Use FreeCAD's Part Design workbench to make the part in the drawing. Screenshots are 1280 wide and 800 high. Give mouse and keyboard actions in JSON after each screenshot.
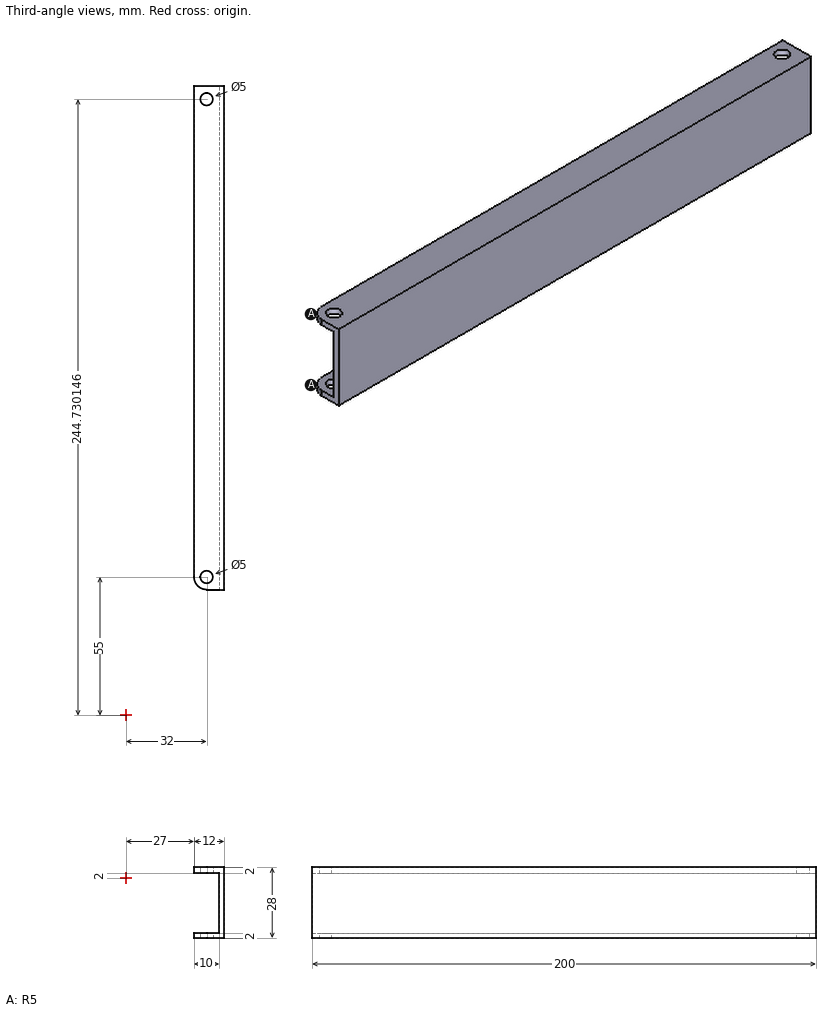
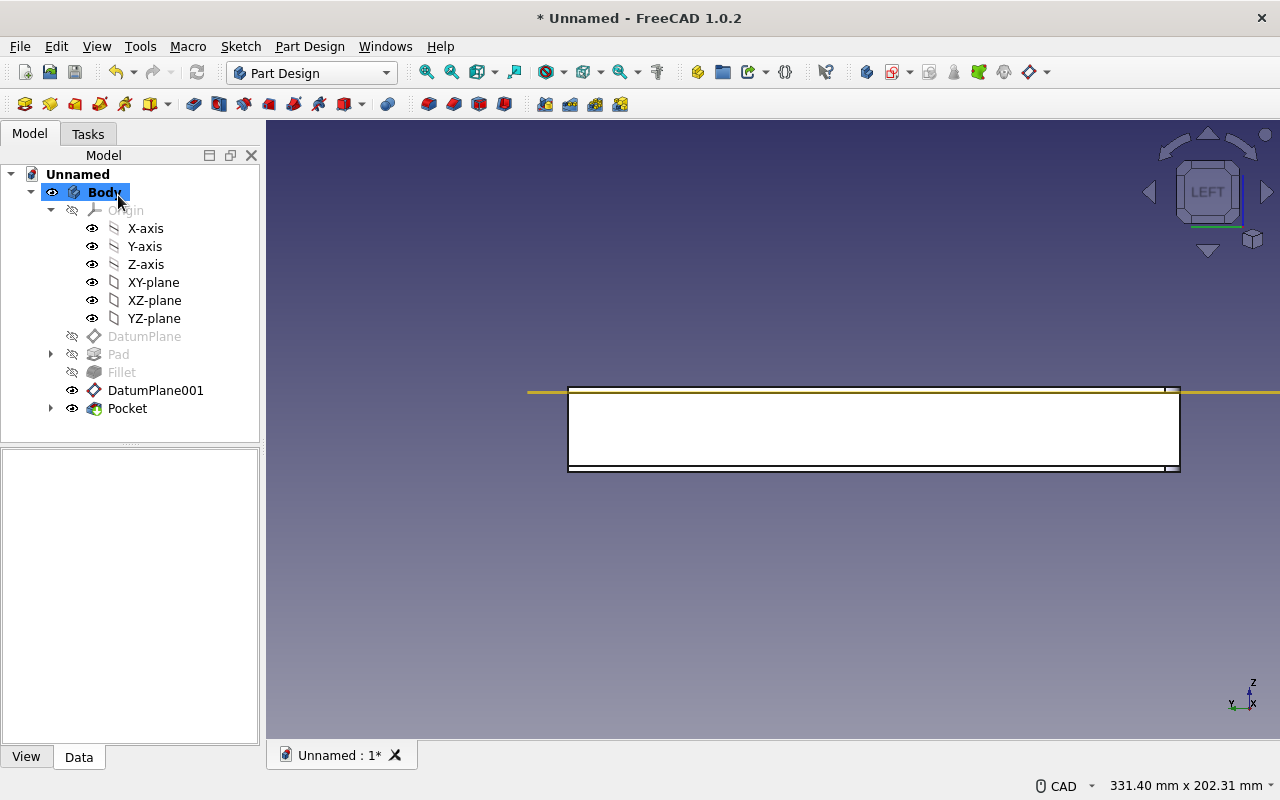
{"action": "left_click", "coordinate": [117, 390]}
{"action": "key", "text": "space"}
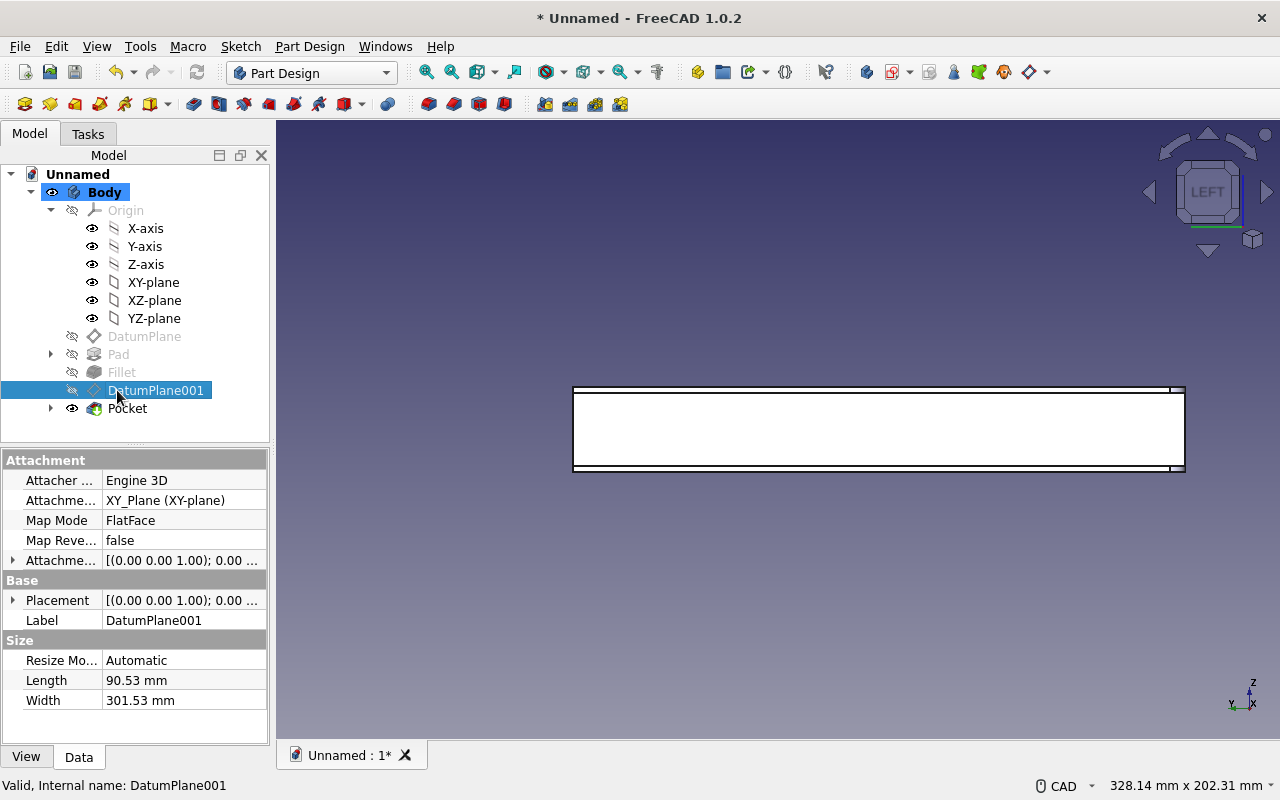
{"action": "left_click", "coordinate": [137, 282]}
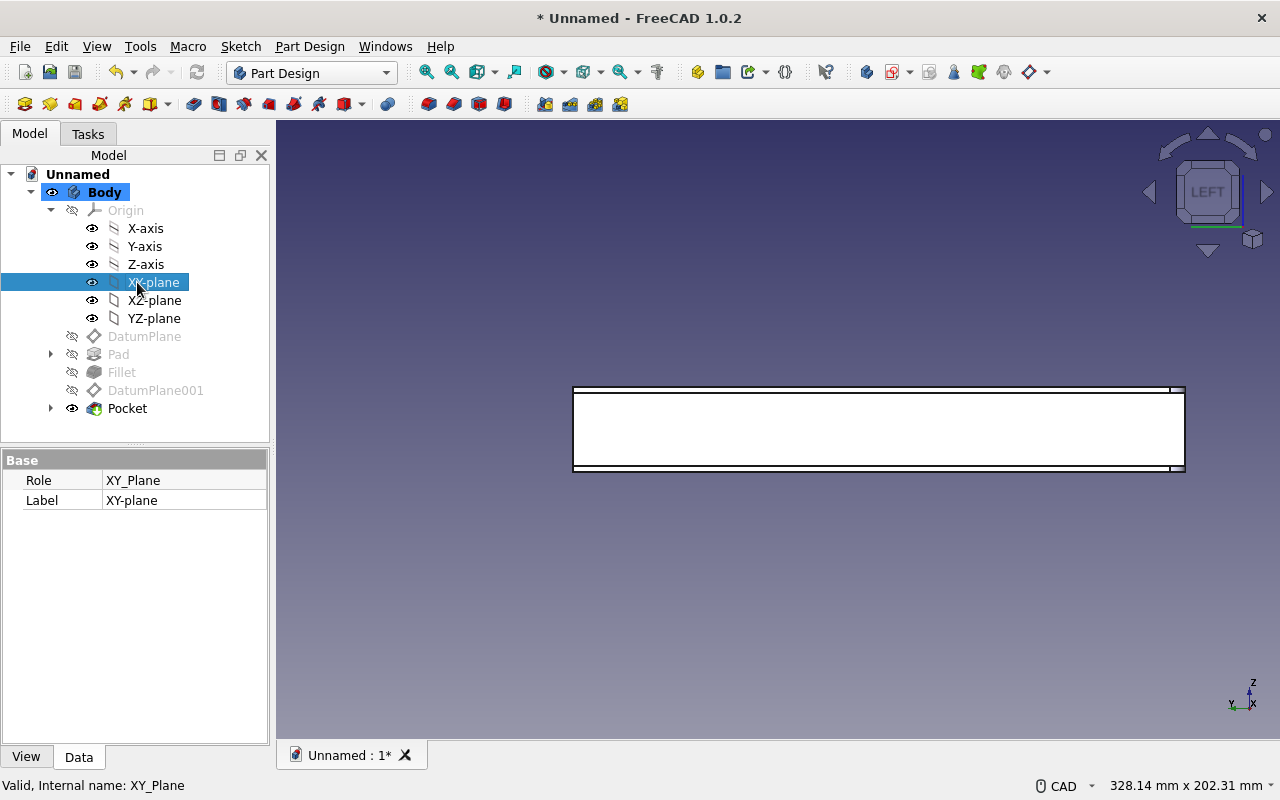
{"action": "left_click", "coordinate": [1028, 72]}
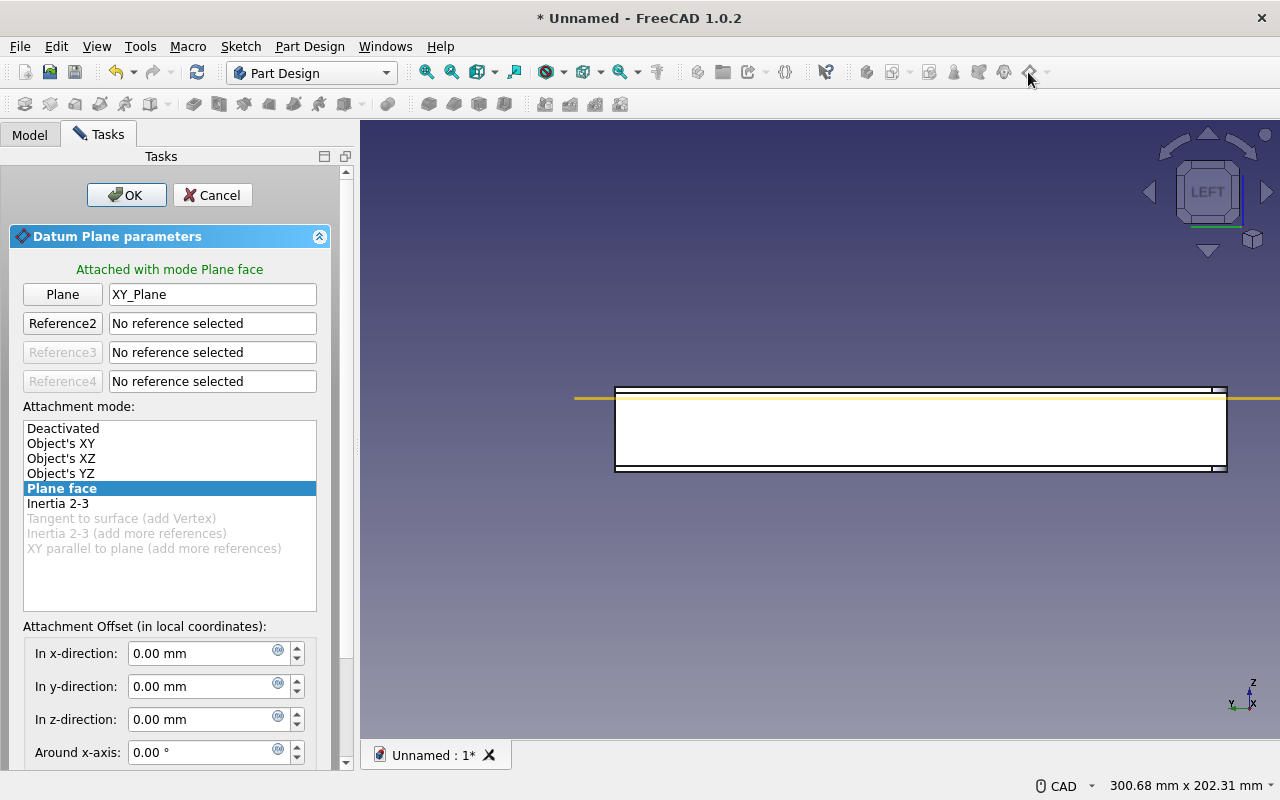
{"action": "triple_click", "coordinate": [210, 720]}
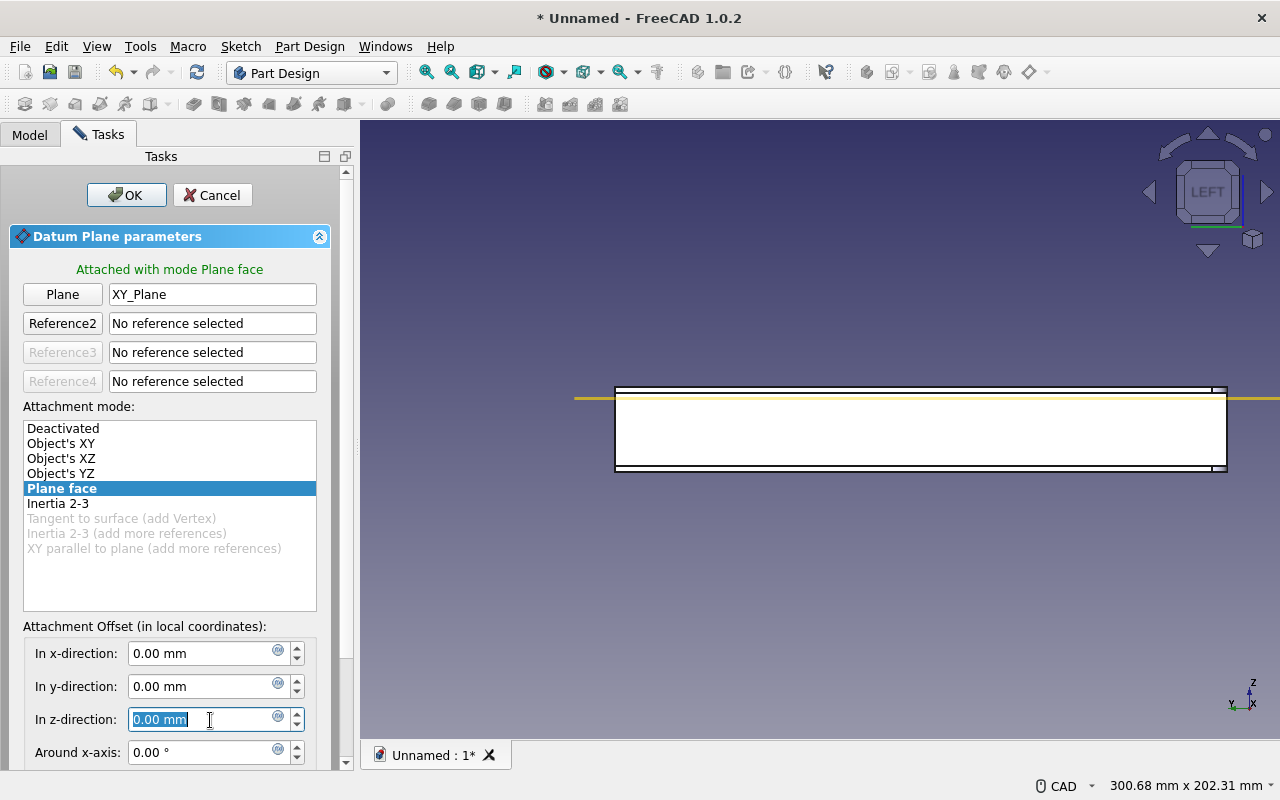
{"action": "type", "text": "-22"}
{"action": "key", "text": "Tab"}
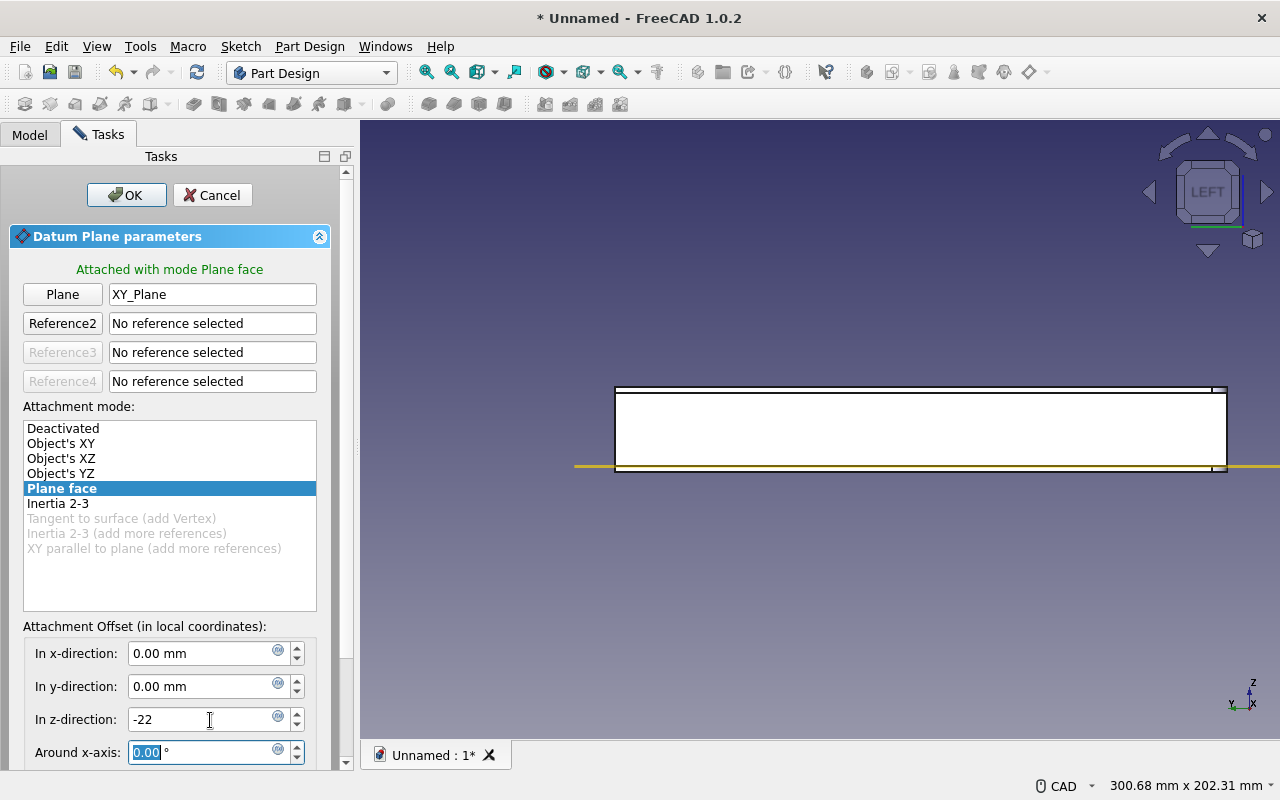
{"action": "left_click", "coordinate": [127, 195]}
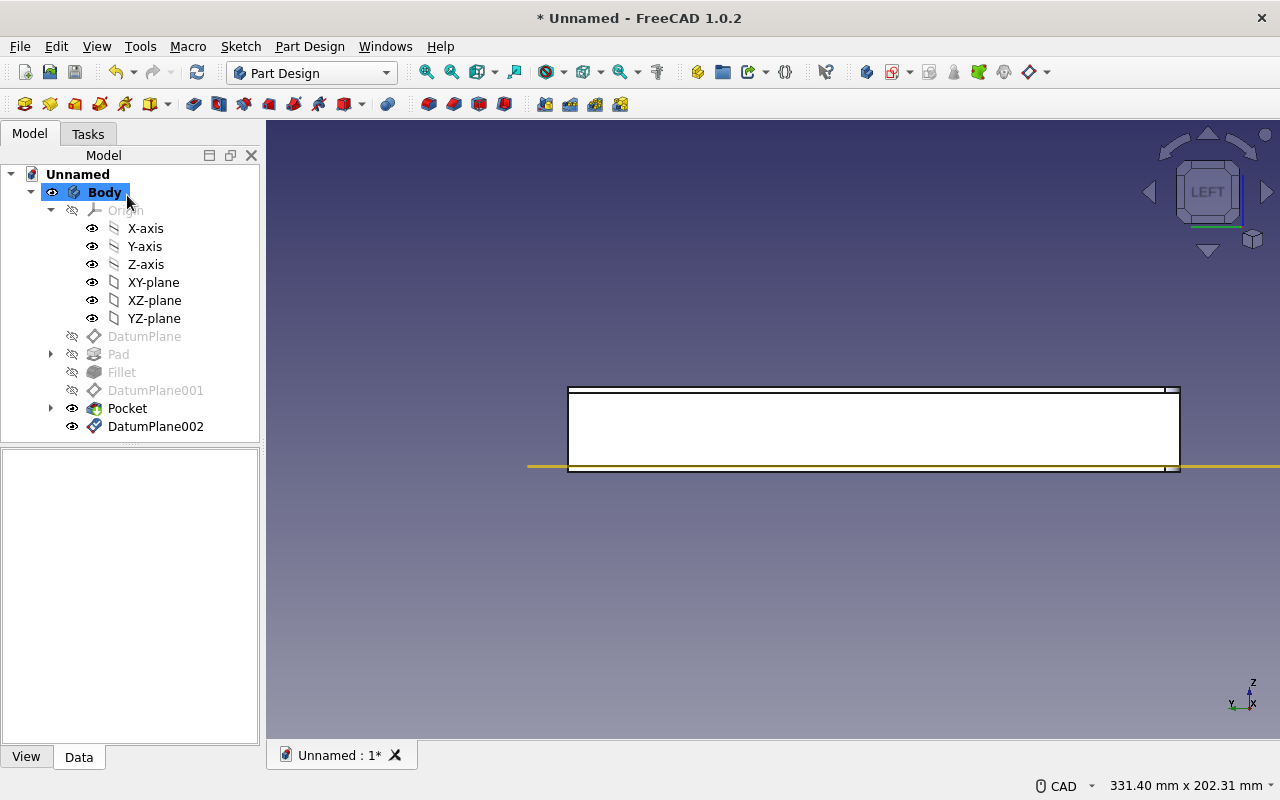
{"action": "left_click", "coordinate": [117, 426]}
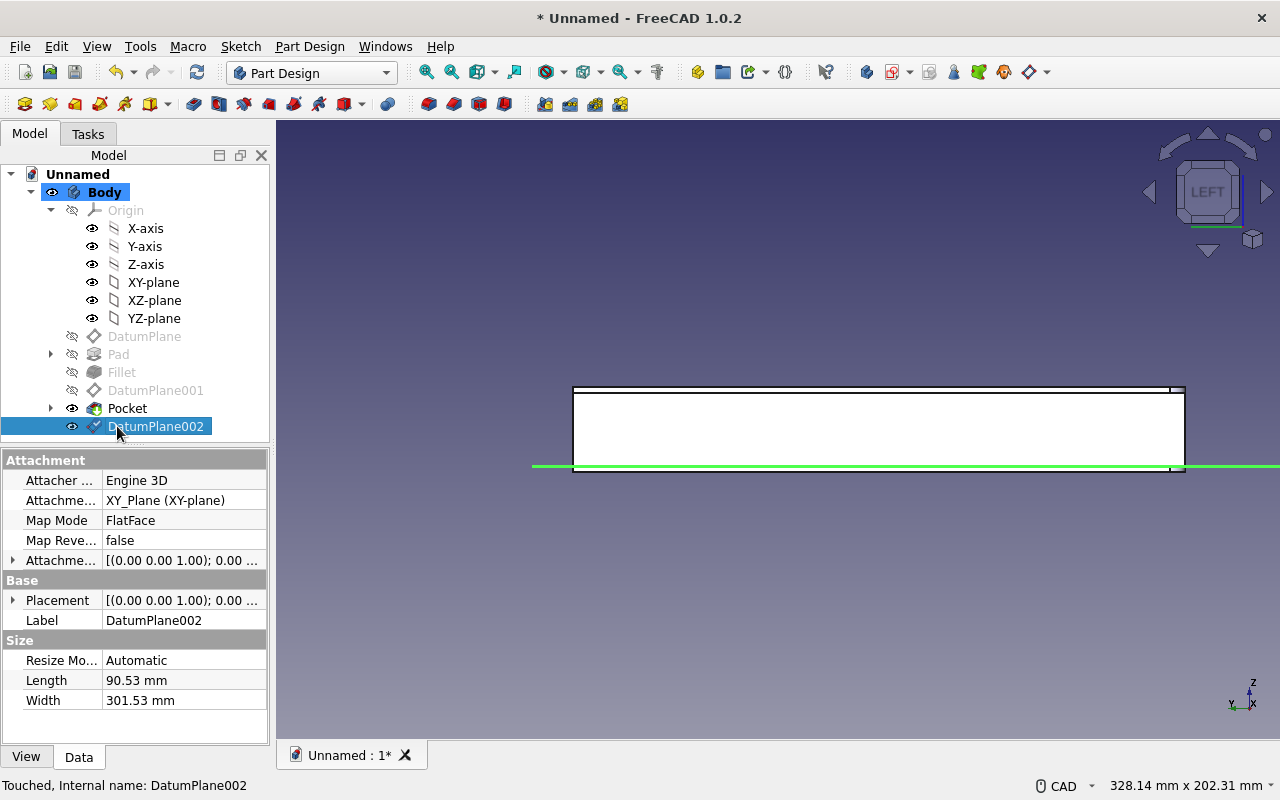
{"action": "left_click", "coordinate": [892, 72]}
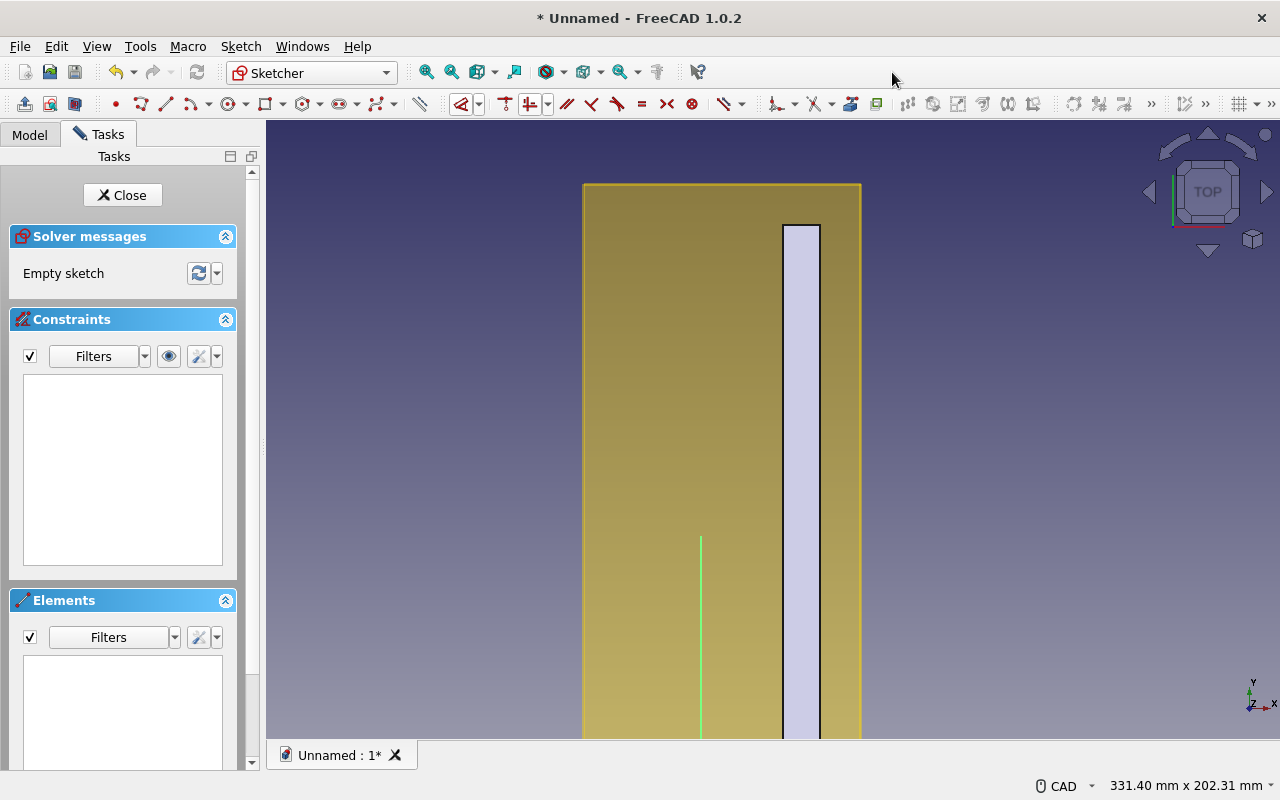
{"action": "left_click", "coordinate": [75, 104]}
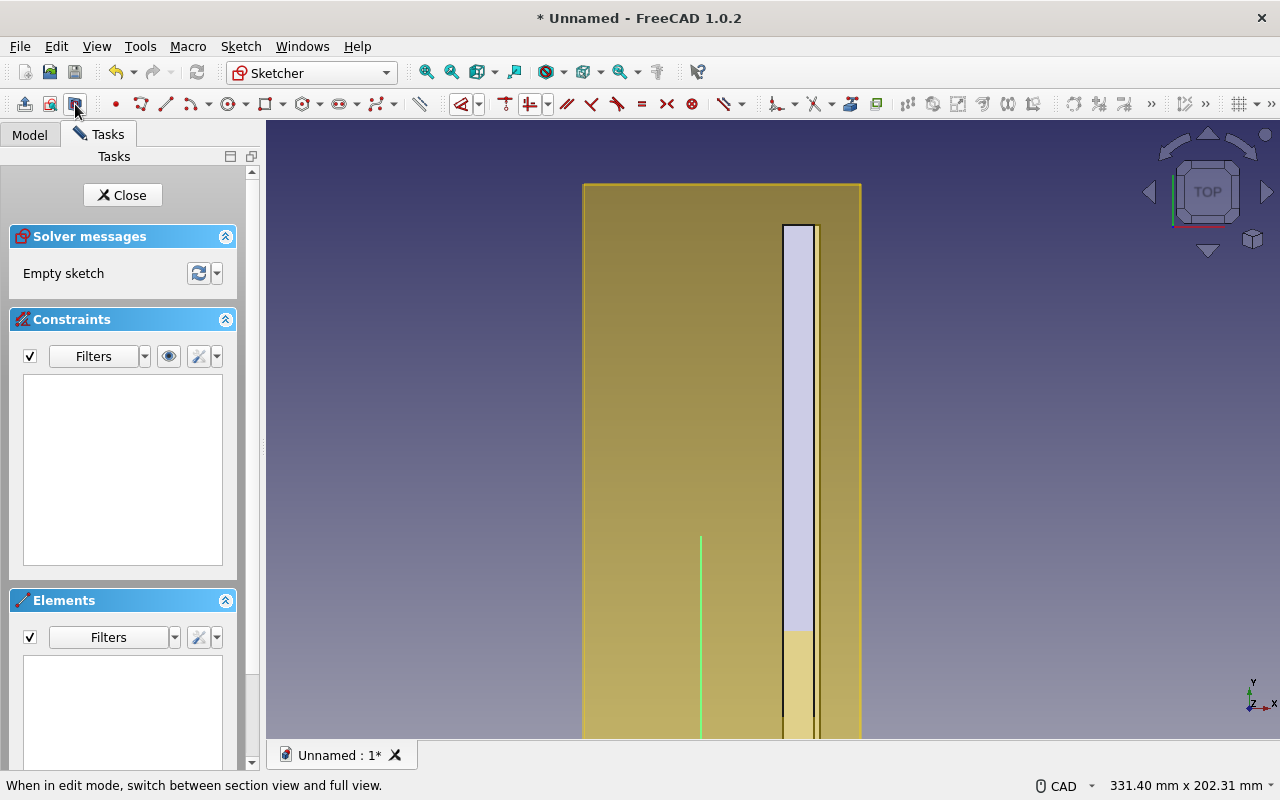
{"action": "scroll", "coordinate": [804, 231], "scroll_direction": "up", "scroll_amount": 15}